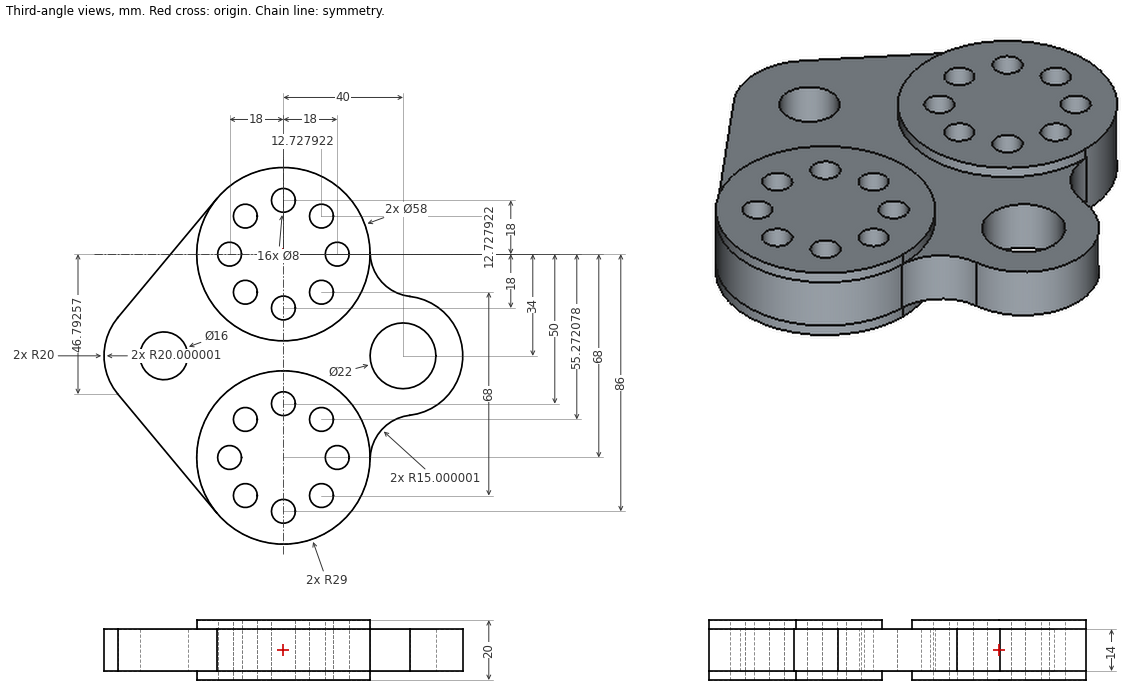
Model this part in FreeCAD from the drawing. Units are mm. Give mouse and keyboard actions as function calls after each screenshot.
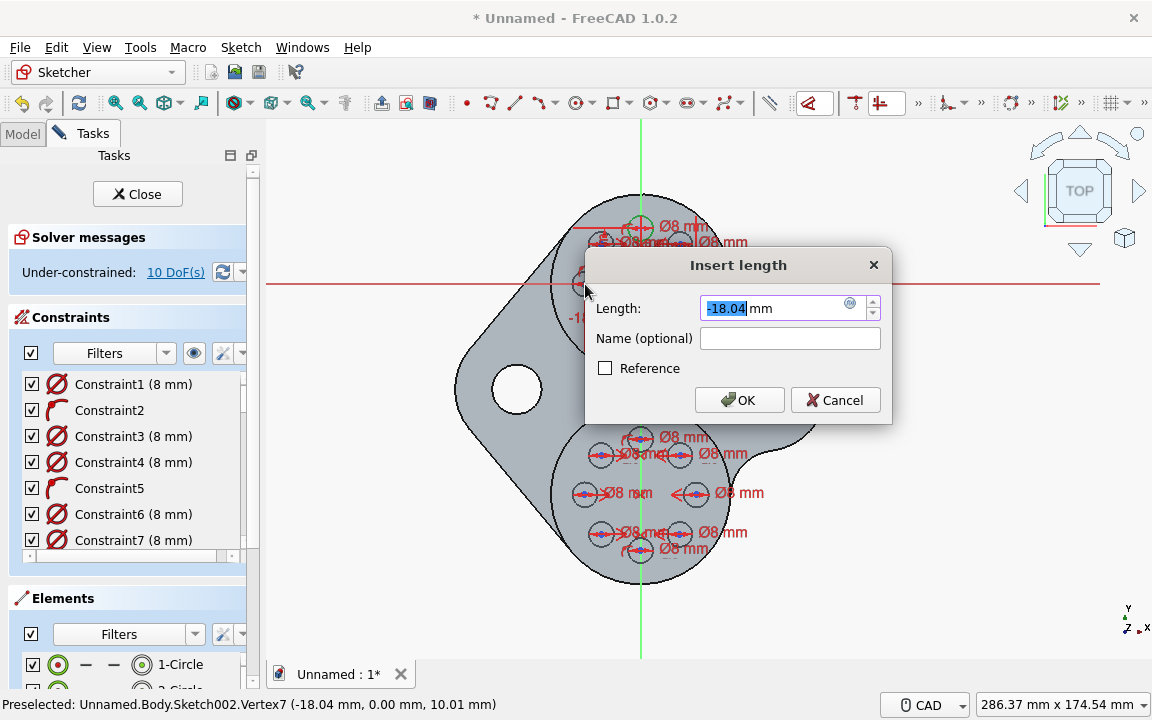
text(-18)
key(Return)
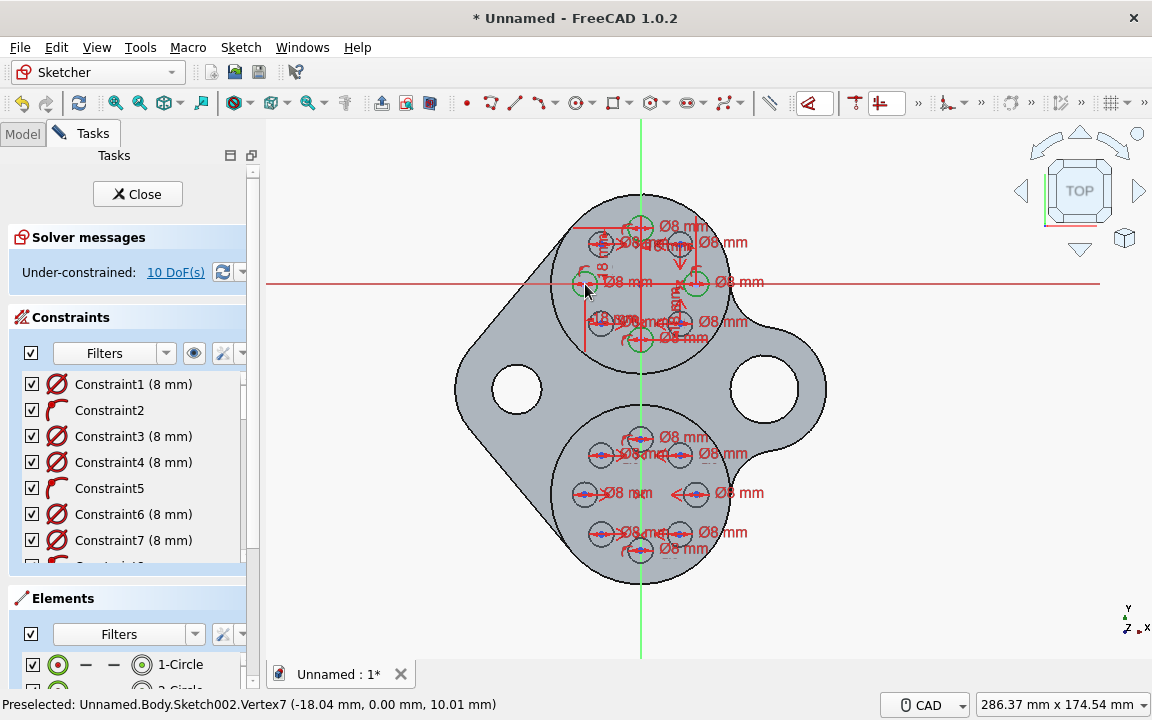
click(641, 439)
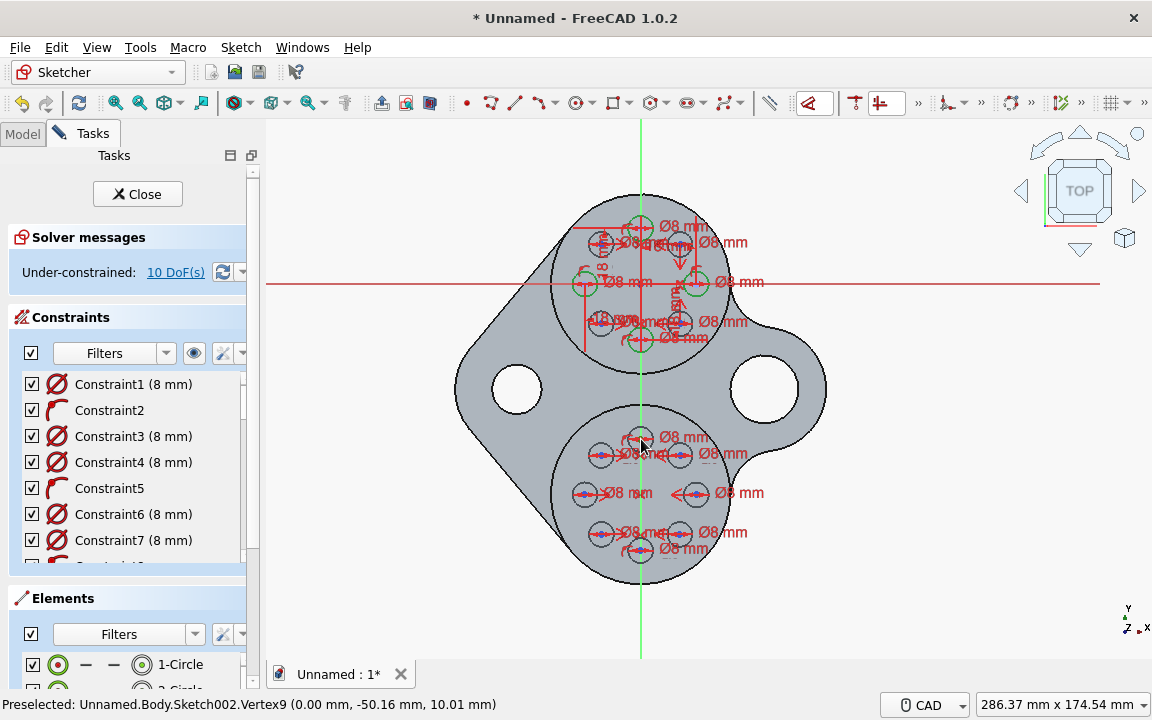
key(i)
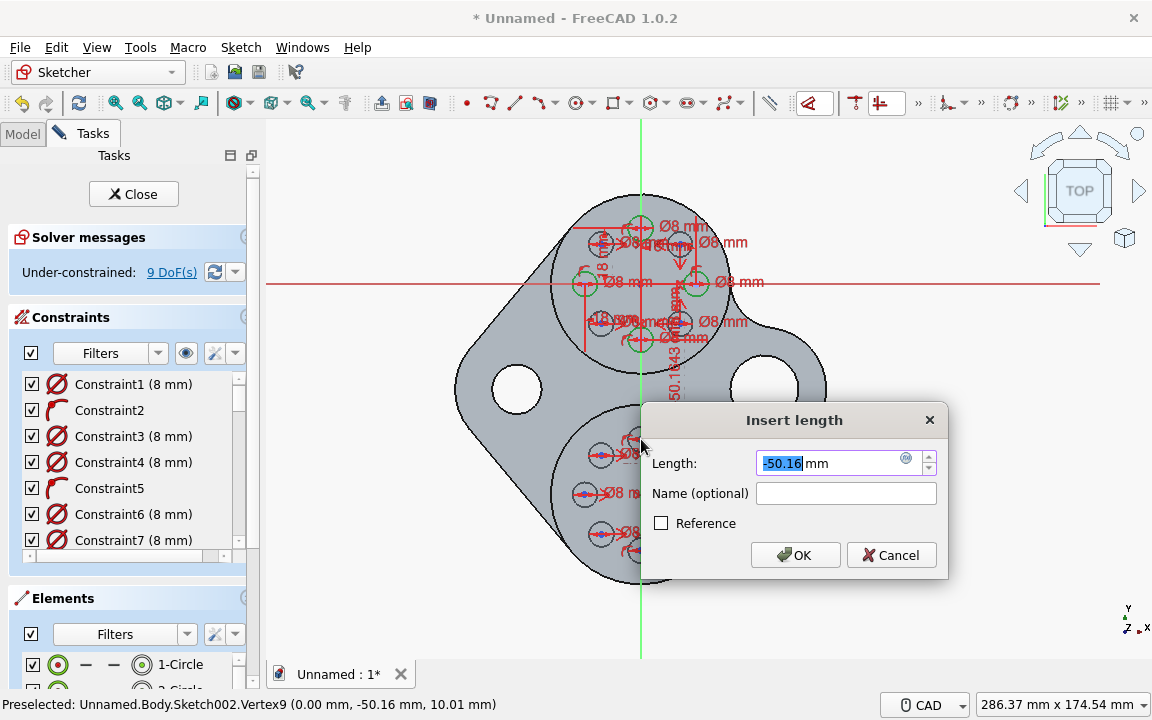
text(-50)
key(Return)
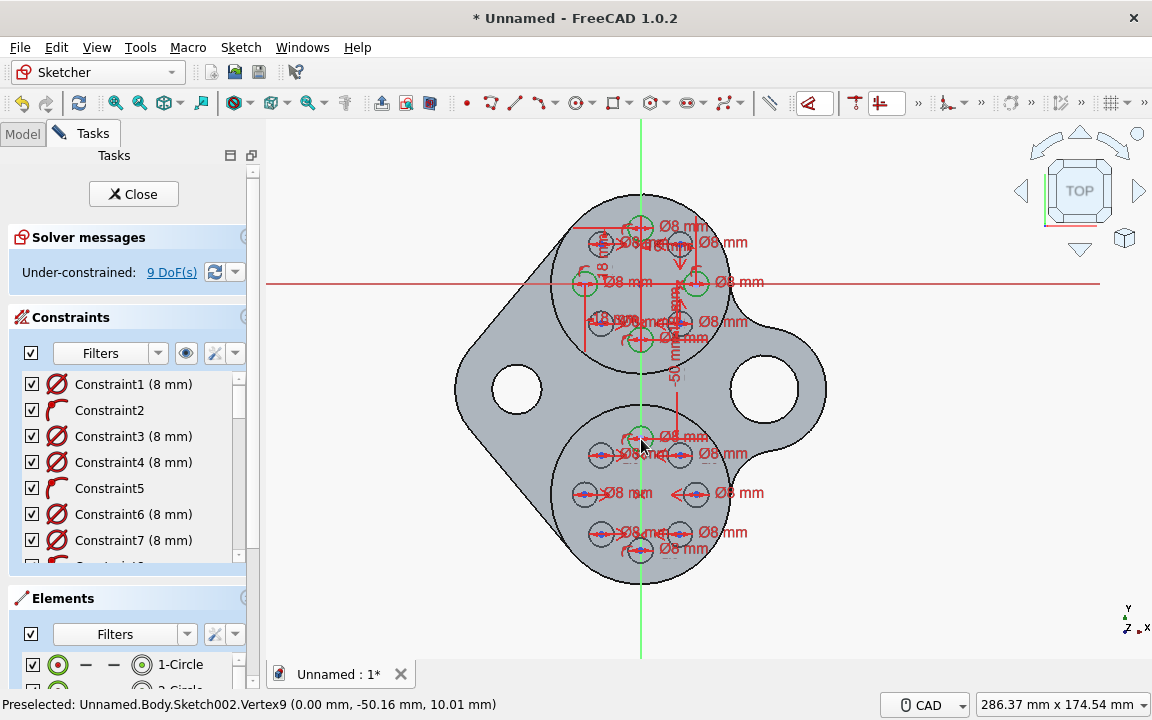
click(696, 495)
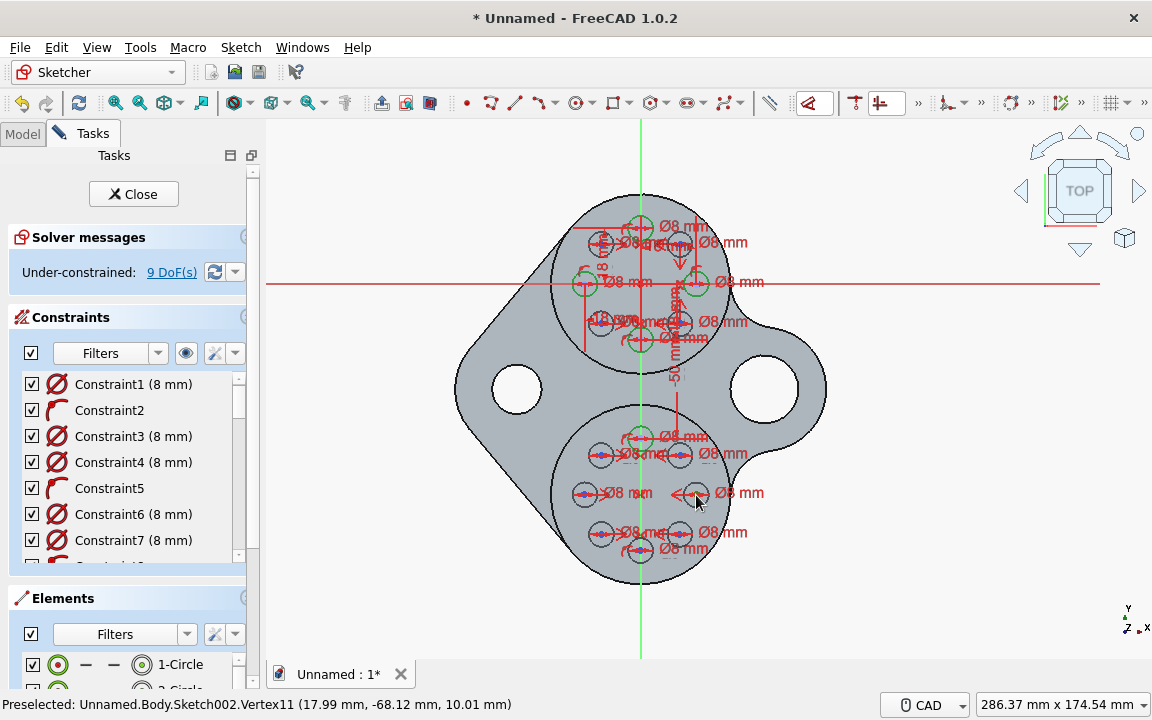
click(828, 104)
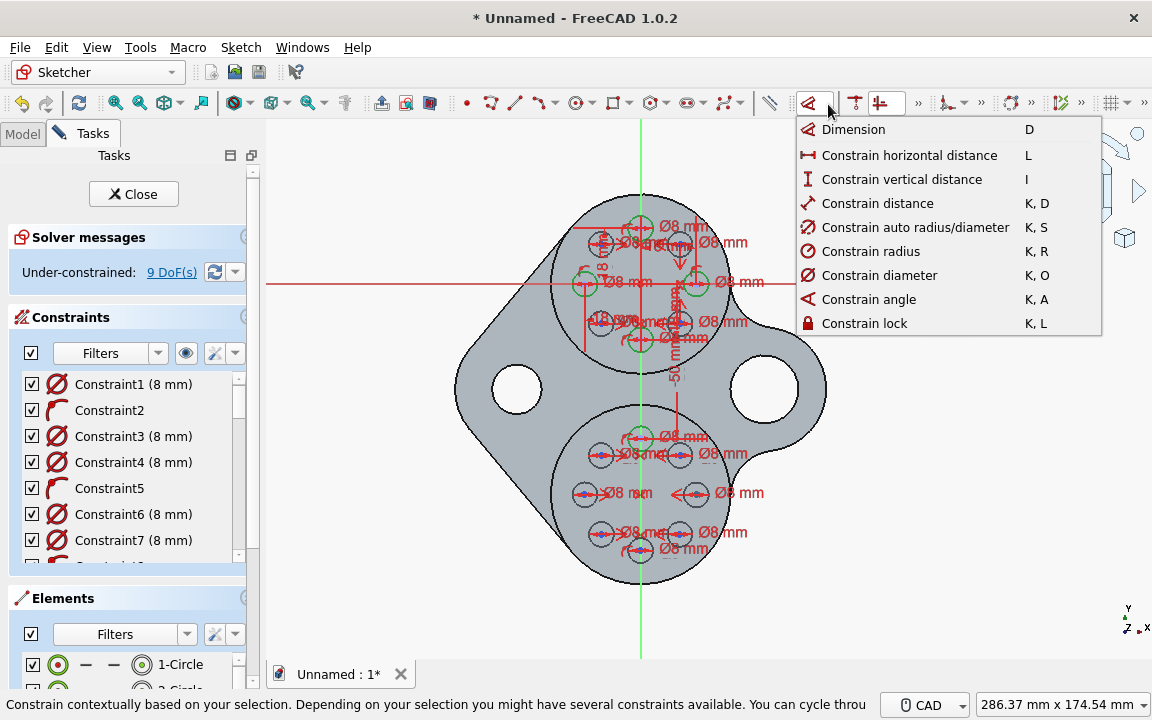
click(949, 155)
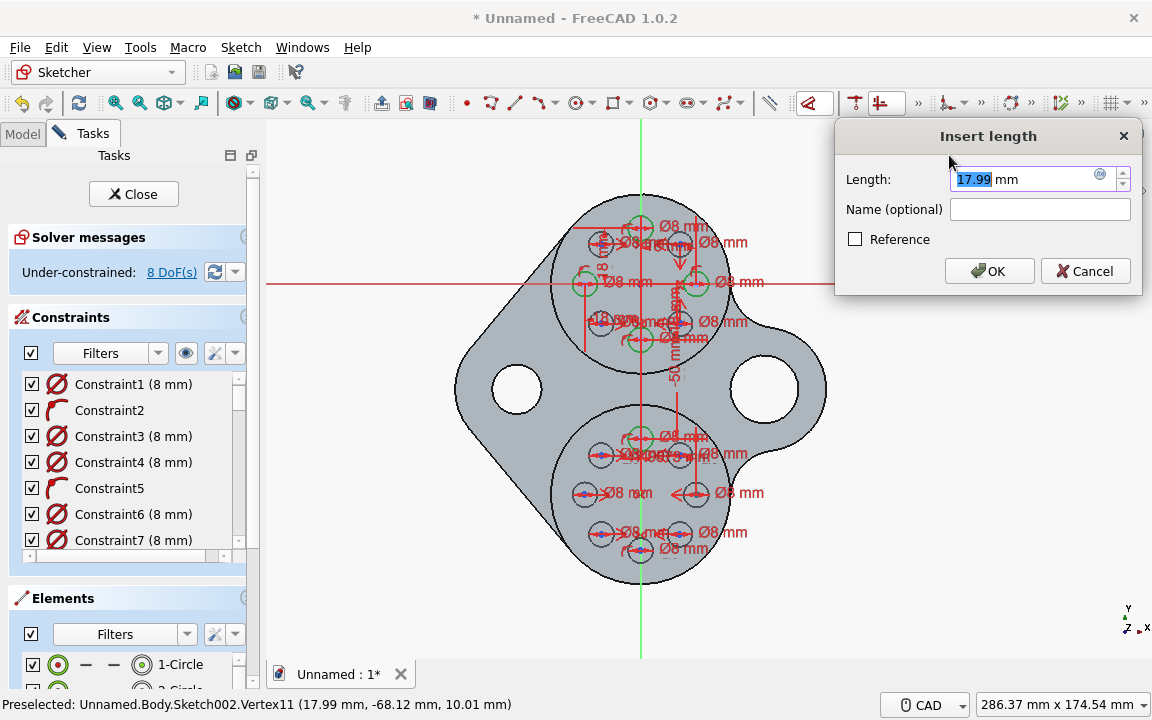
text(18)
key(Return)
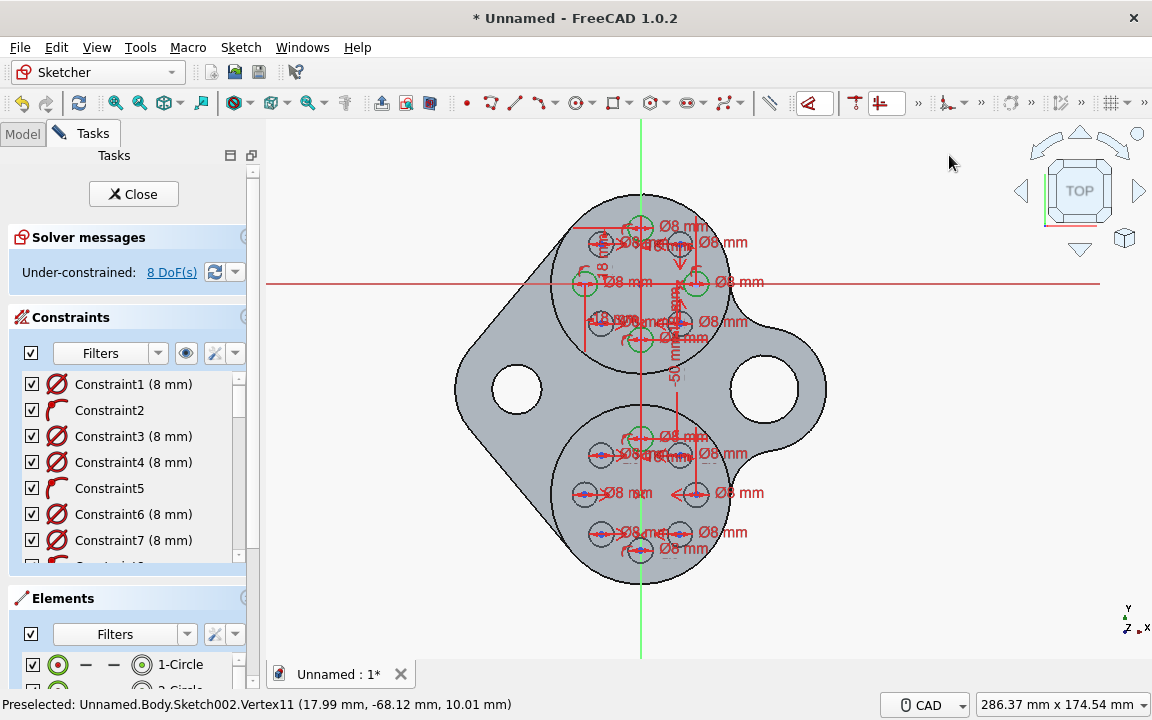
click(696, 495)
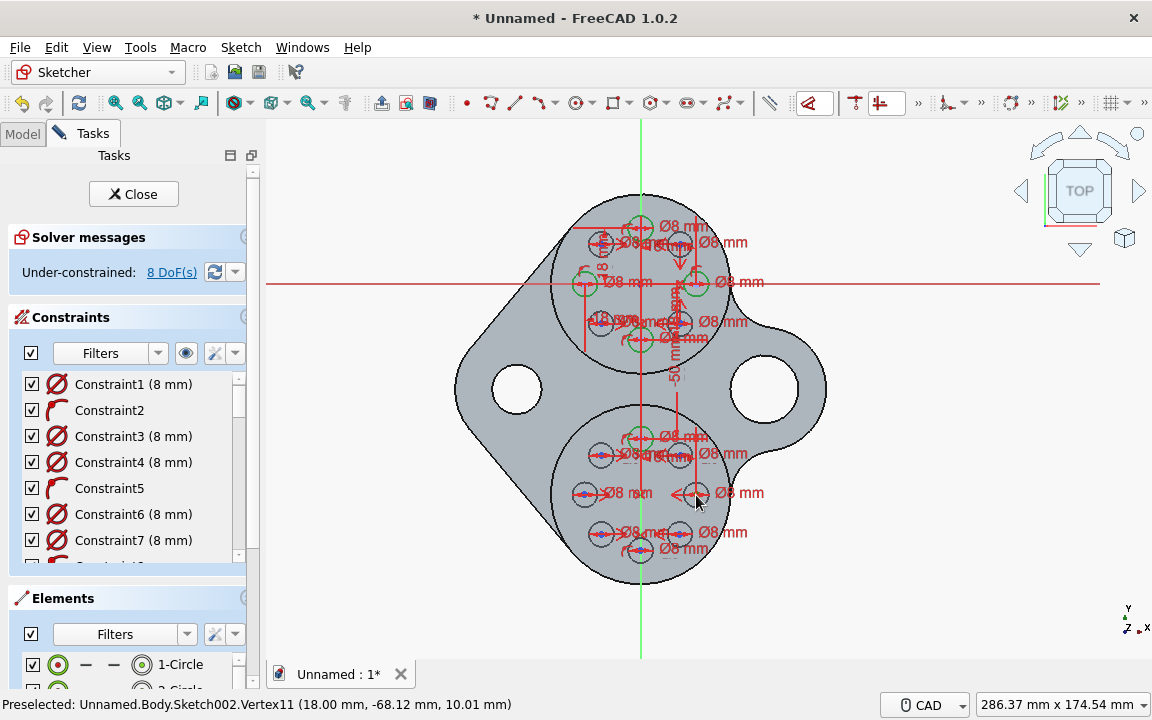
key(i)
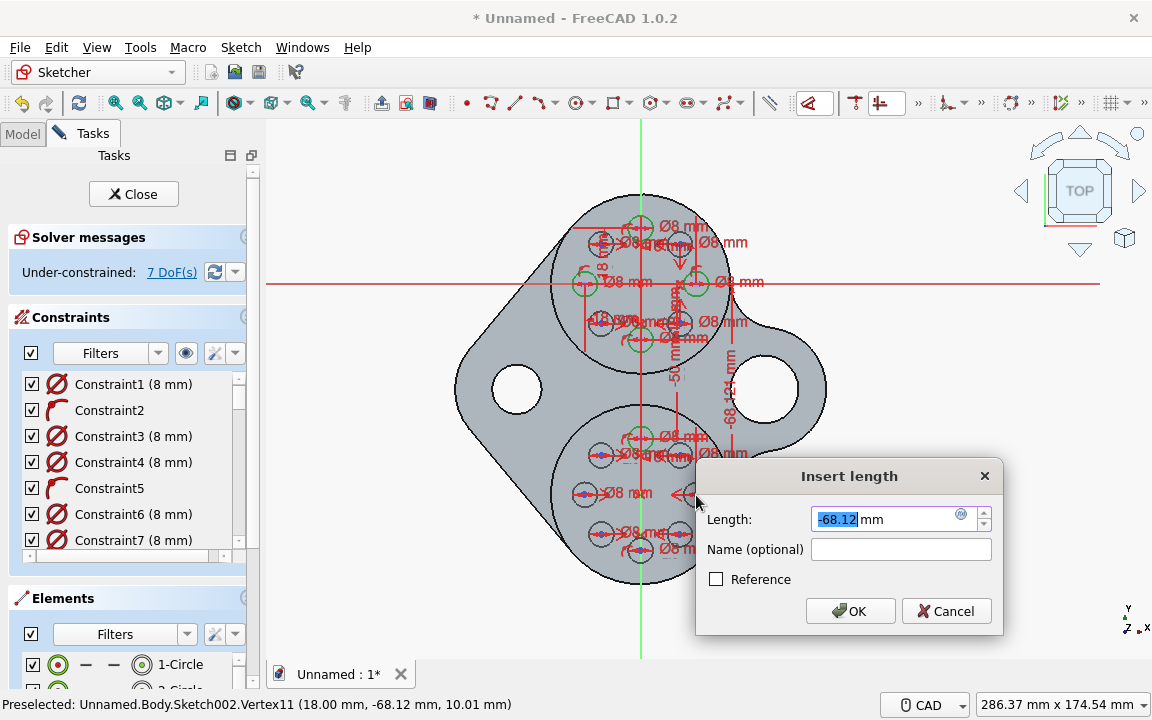
text(-68)
key(Return)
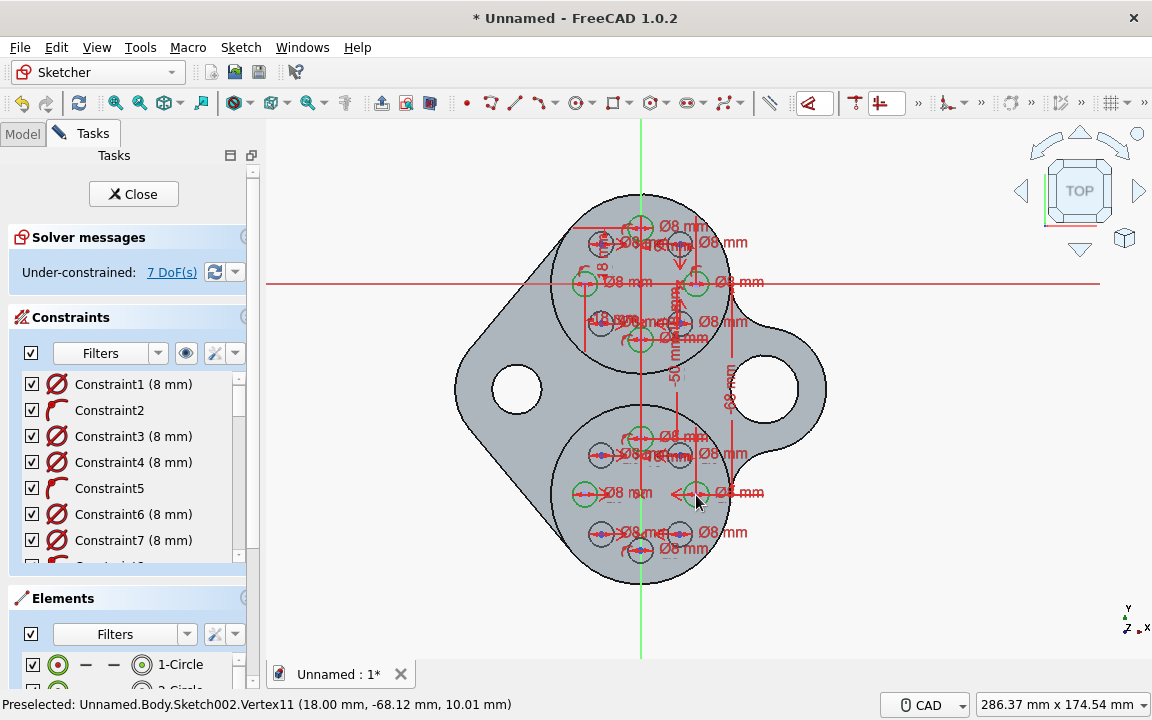
click(641, 551)